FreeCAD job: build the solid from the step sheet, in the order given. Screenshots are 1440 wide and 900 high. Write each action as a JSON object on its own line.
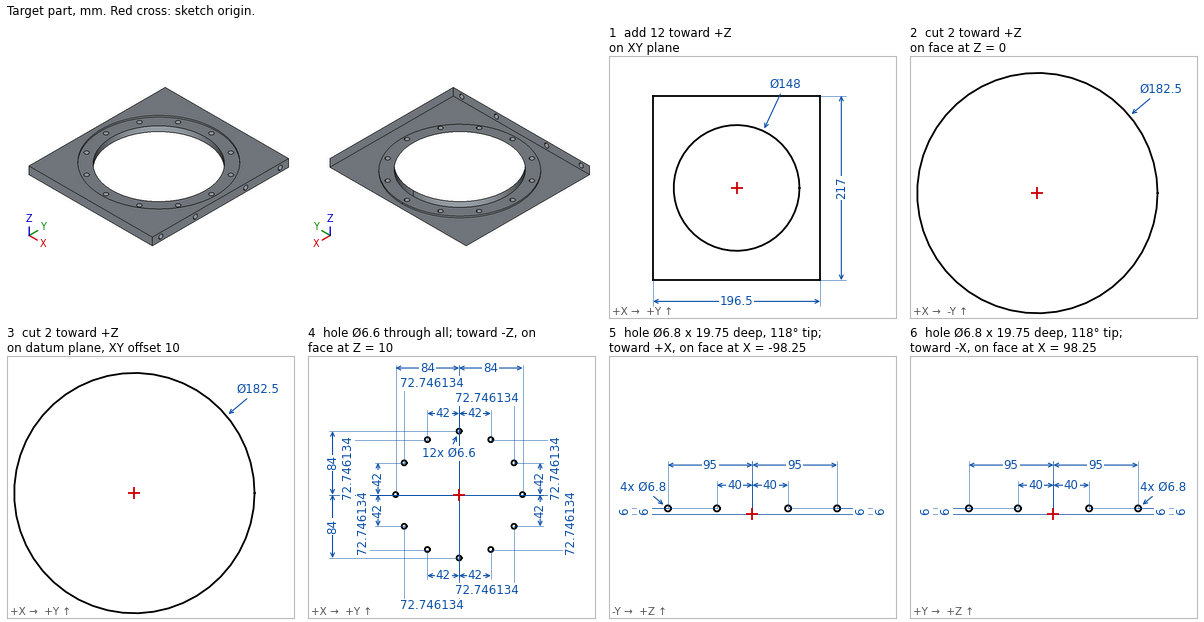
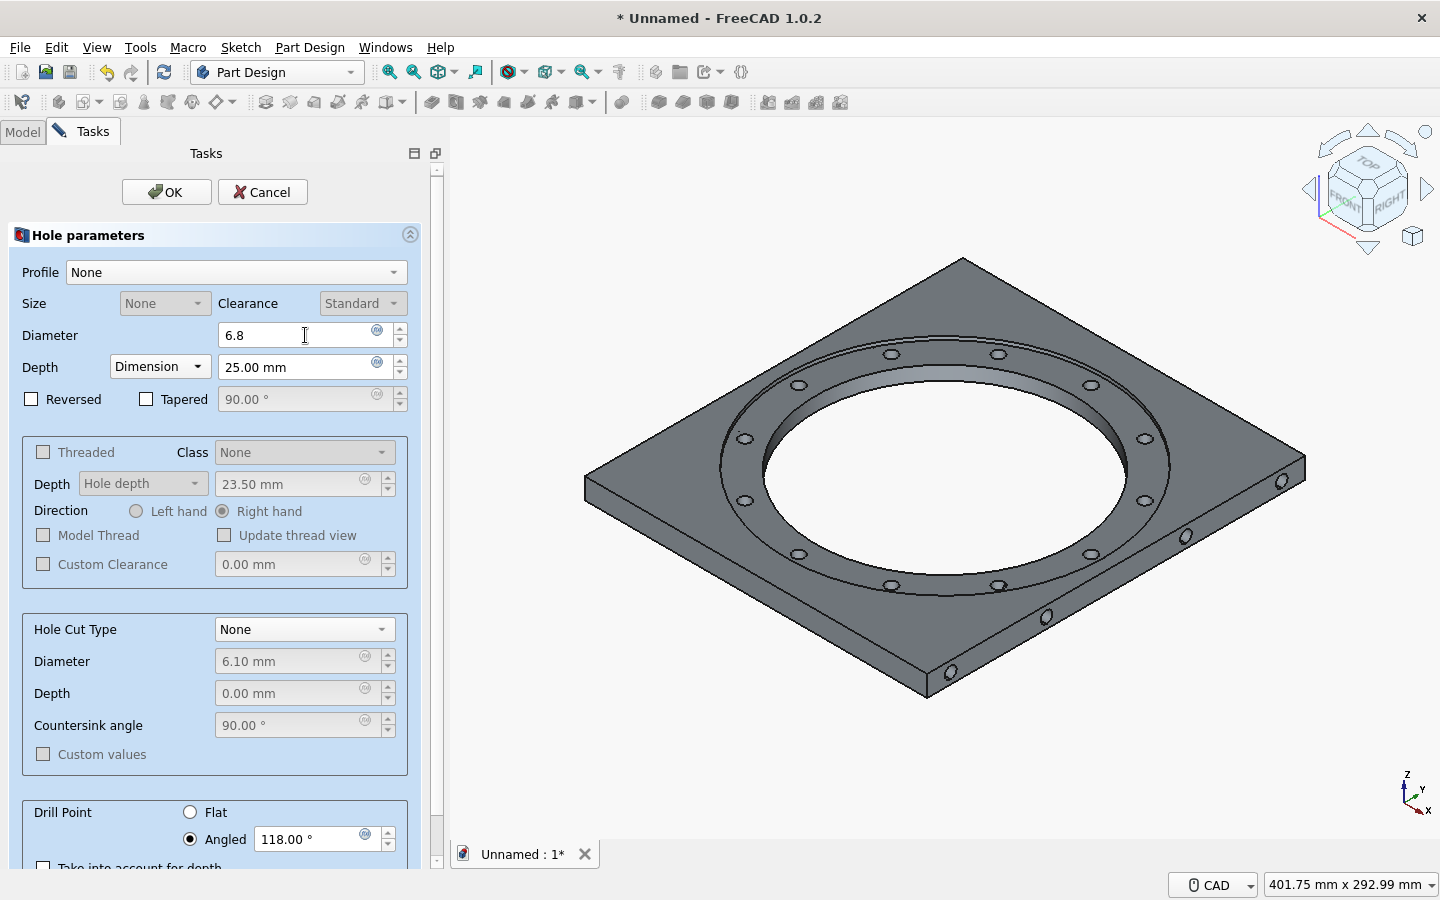
{"action": "triple_click", "coordinate": [305, 367]}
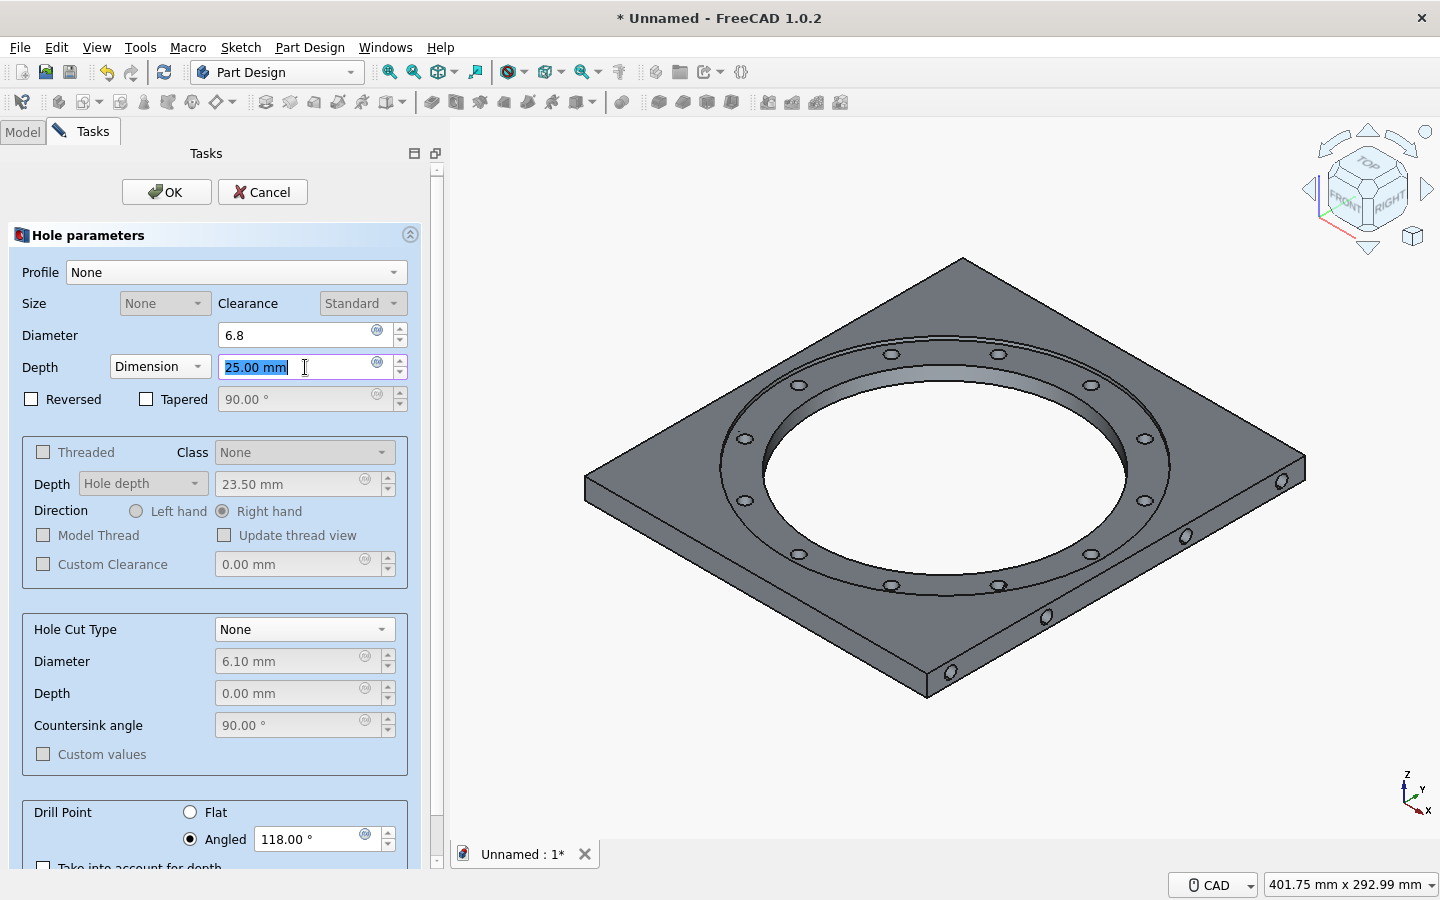
{"action": "type", "text": "19.75"}
{"action": "key", "text": "Tab"}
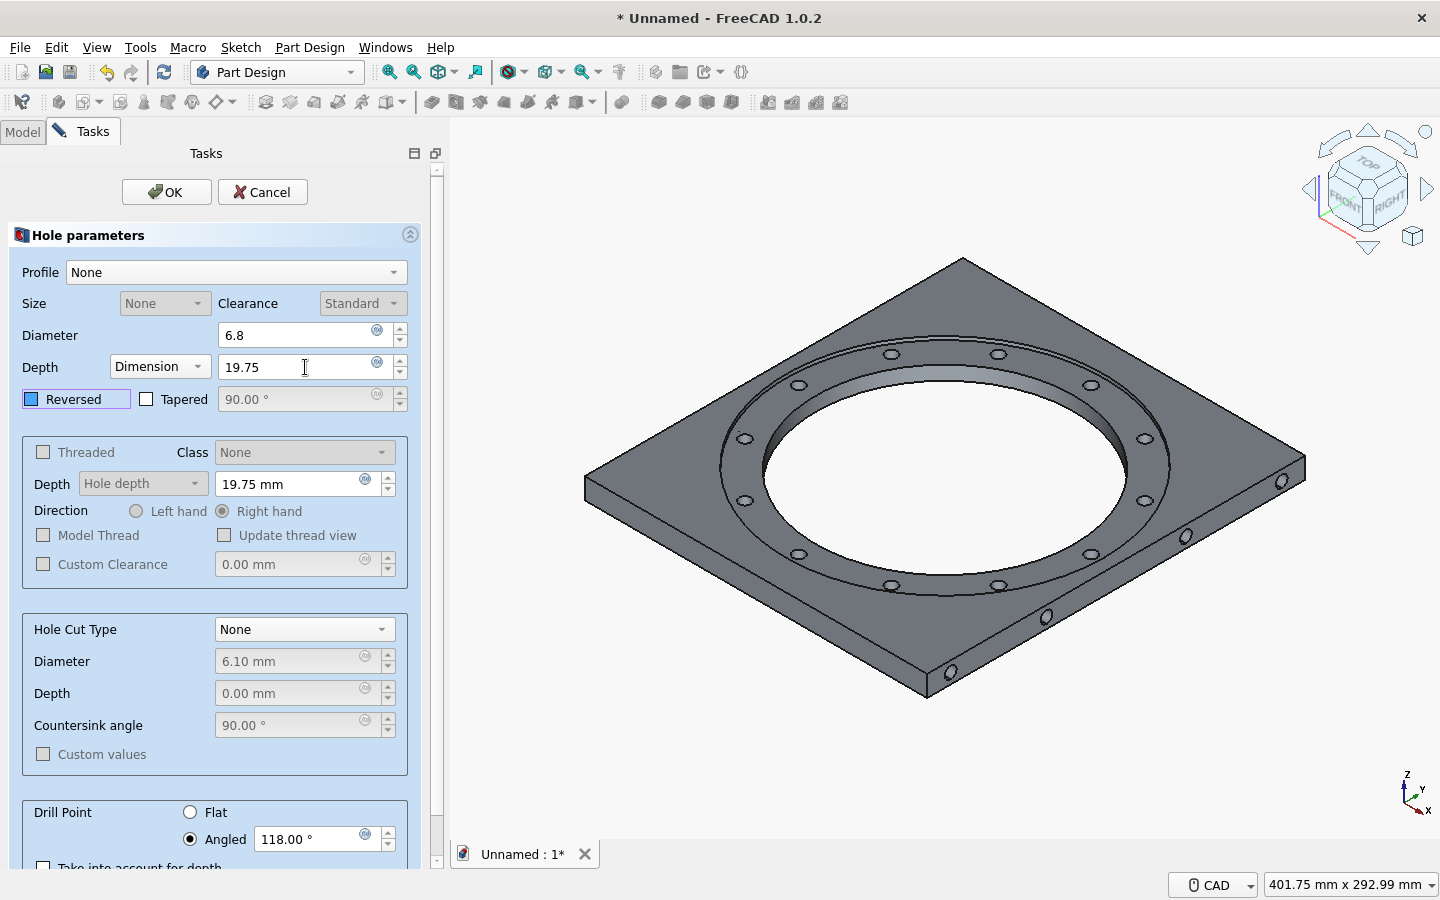
{"action": "left_click", "coordinate": [167, 192]}